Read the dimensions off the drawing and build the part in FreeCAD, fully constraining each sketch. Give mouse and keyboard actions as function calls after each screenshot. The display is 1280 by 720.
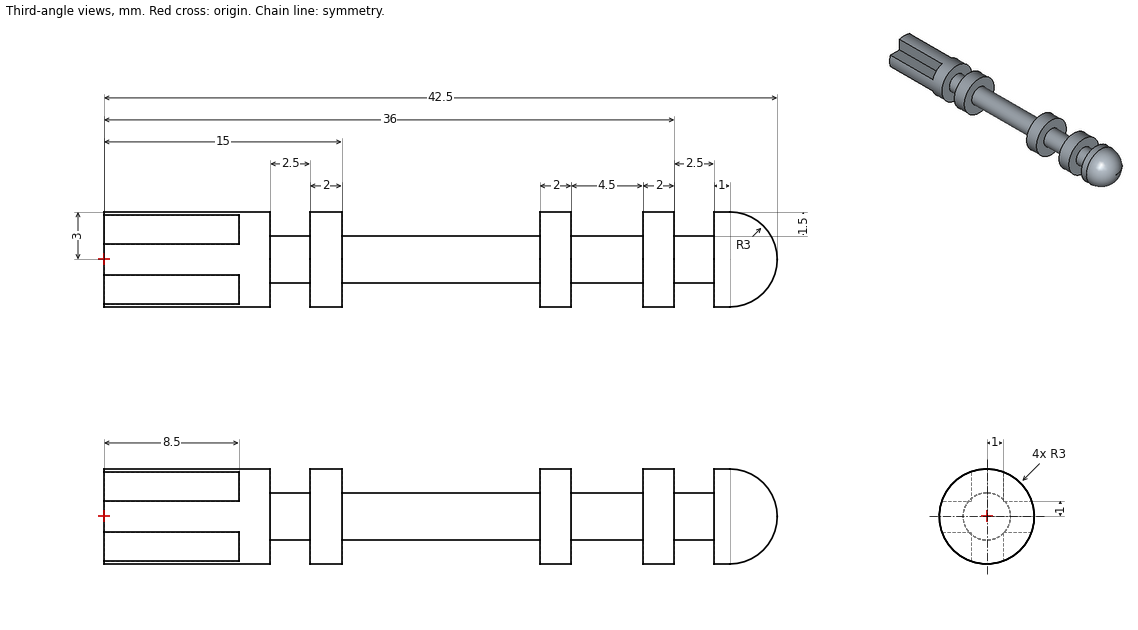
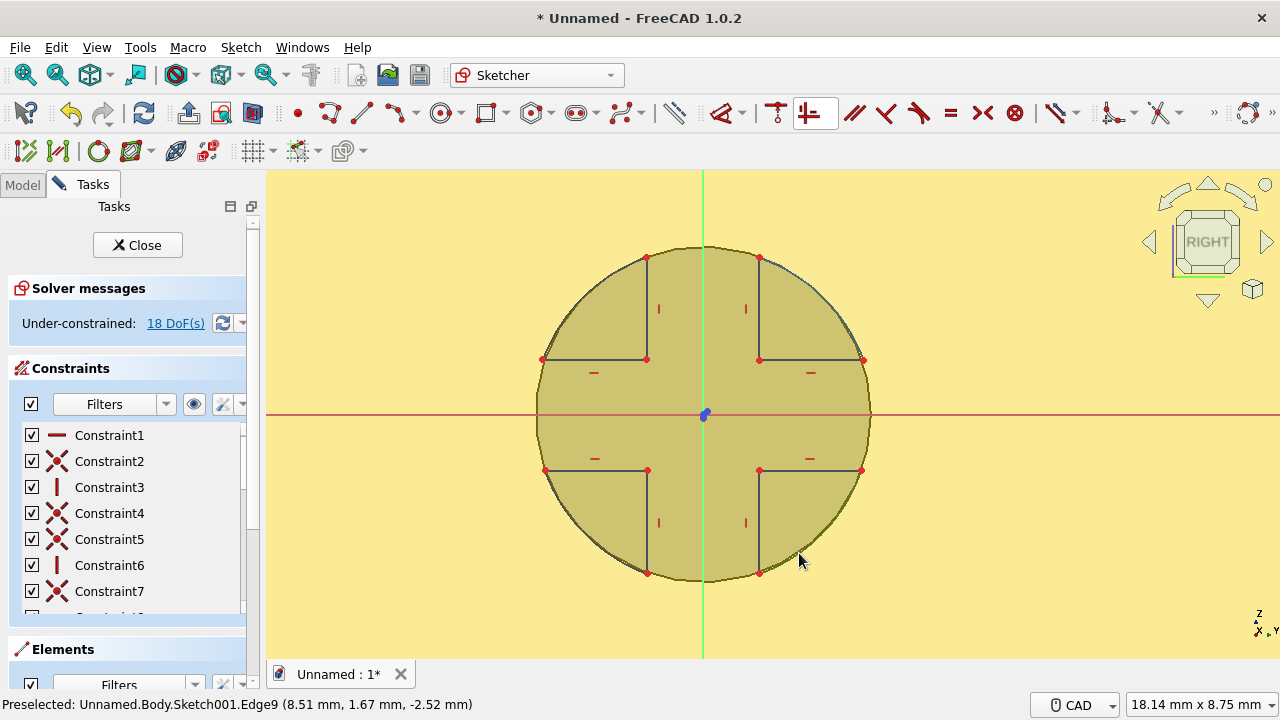
click(776, 114)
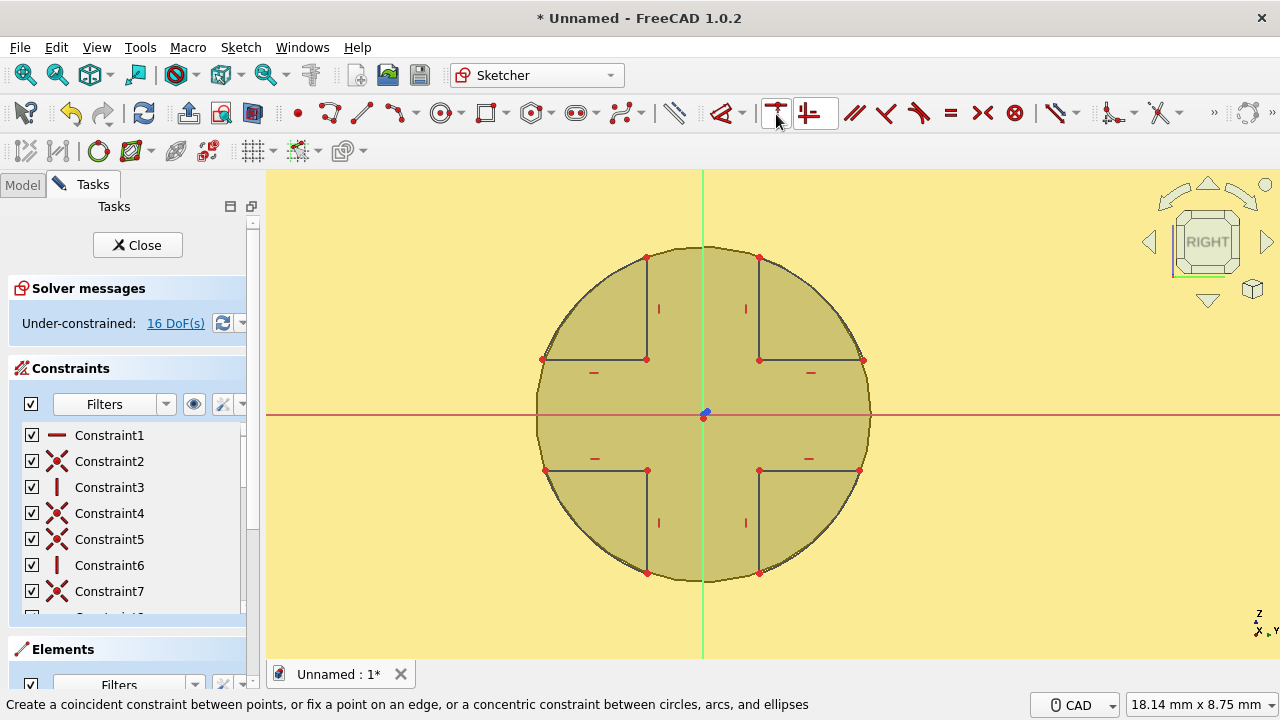
click(842, 320)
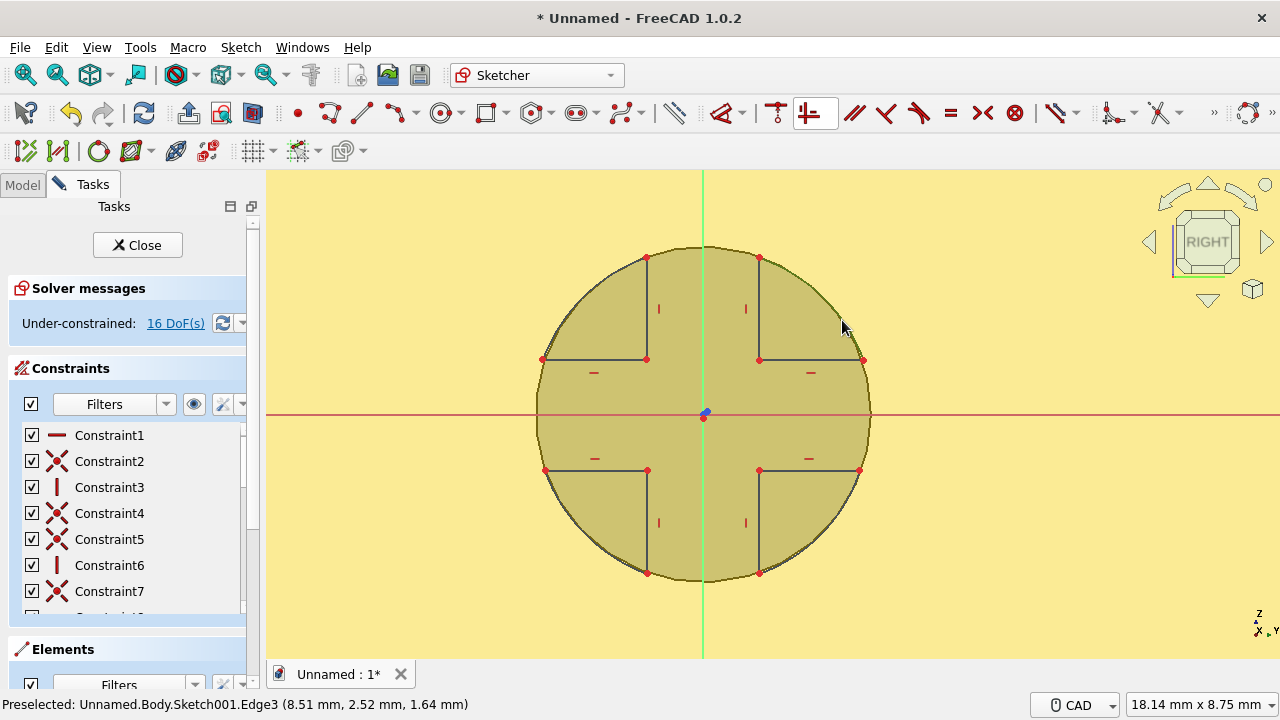
click(566, 511)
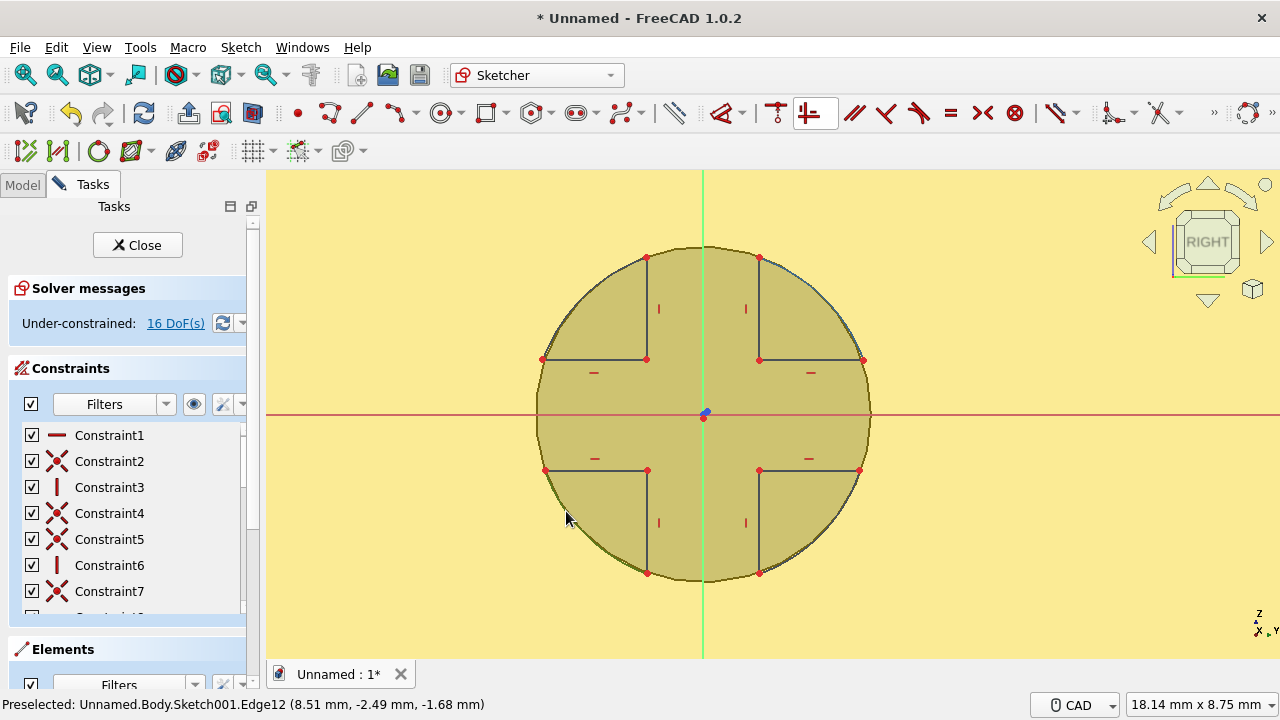
click(776, 114)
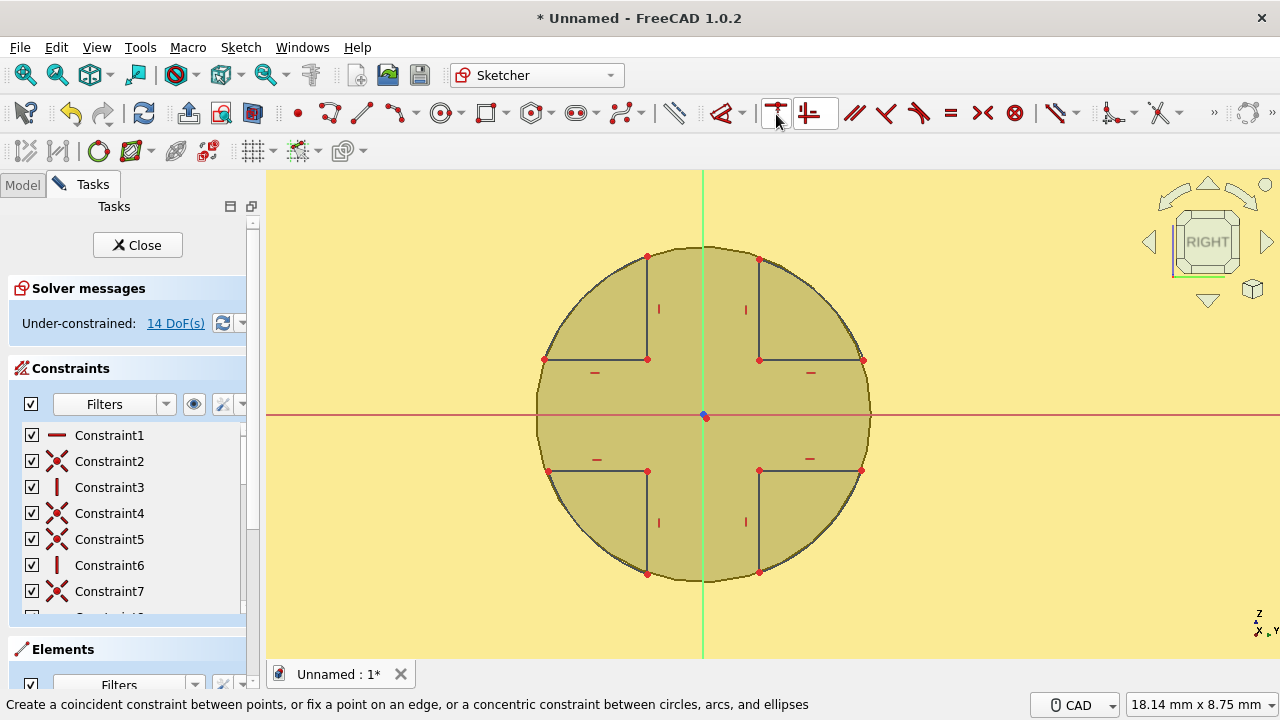
drag(693, 404, 717, 428)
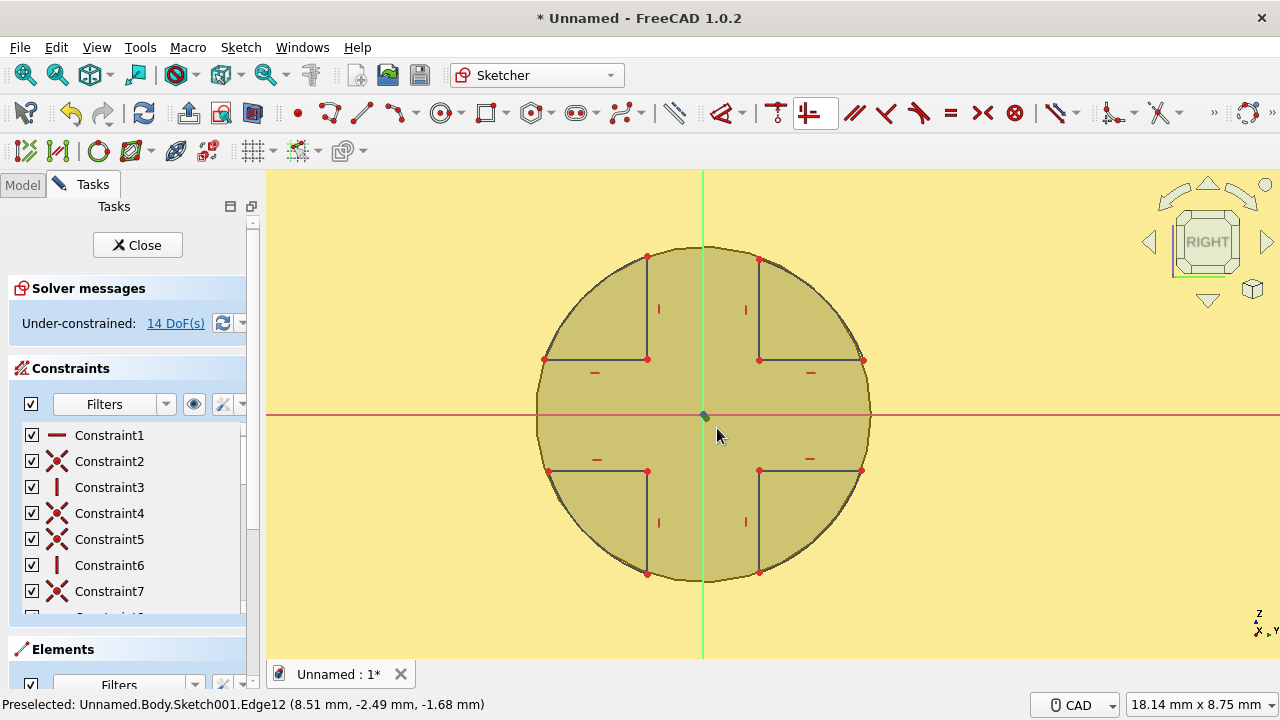
click(776, 114)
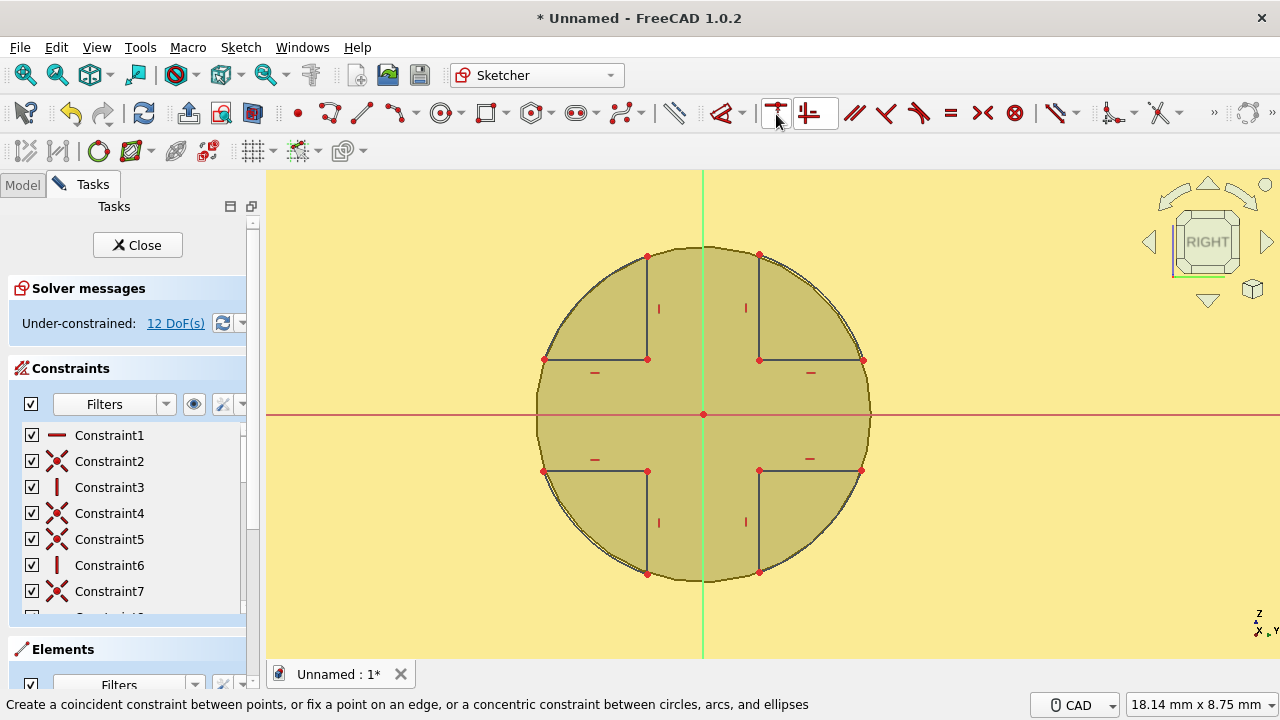
click(843, 319)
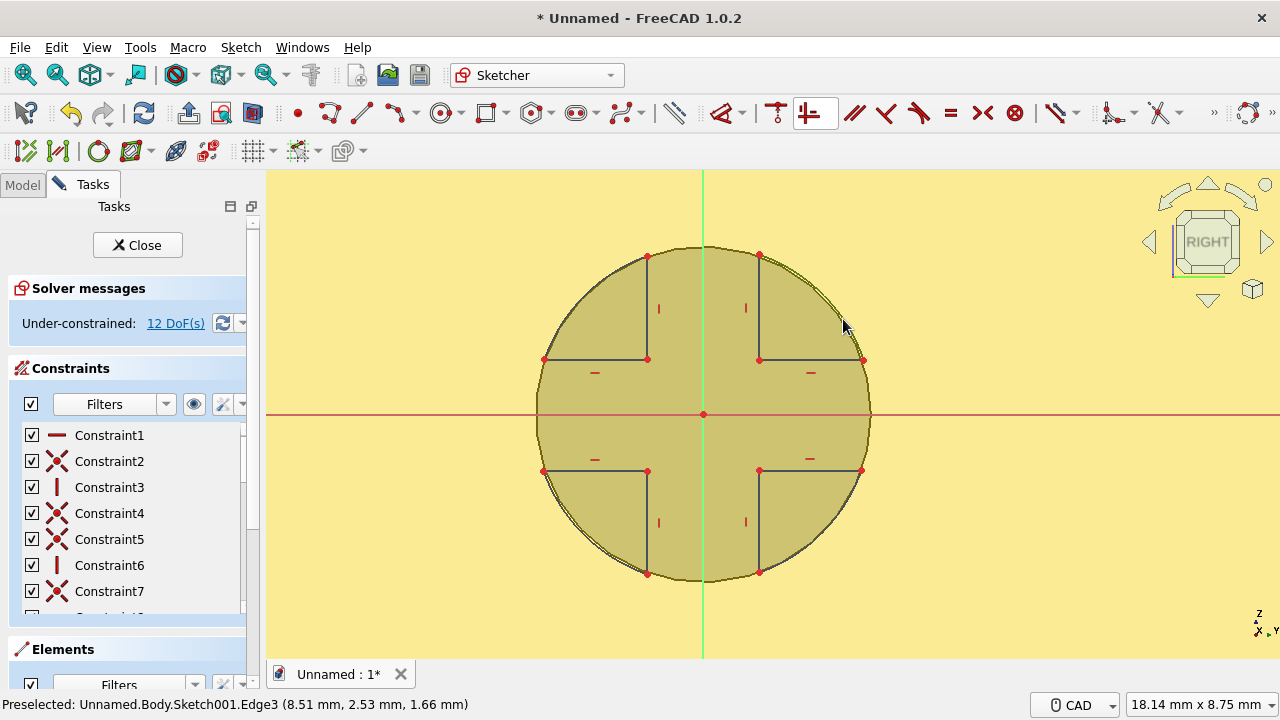
click(607, 277)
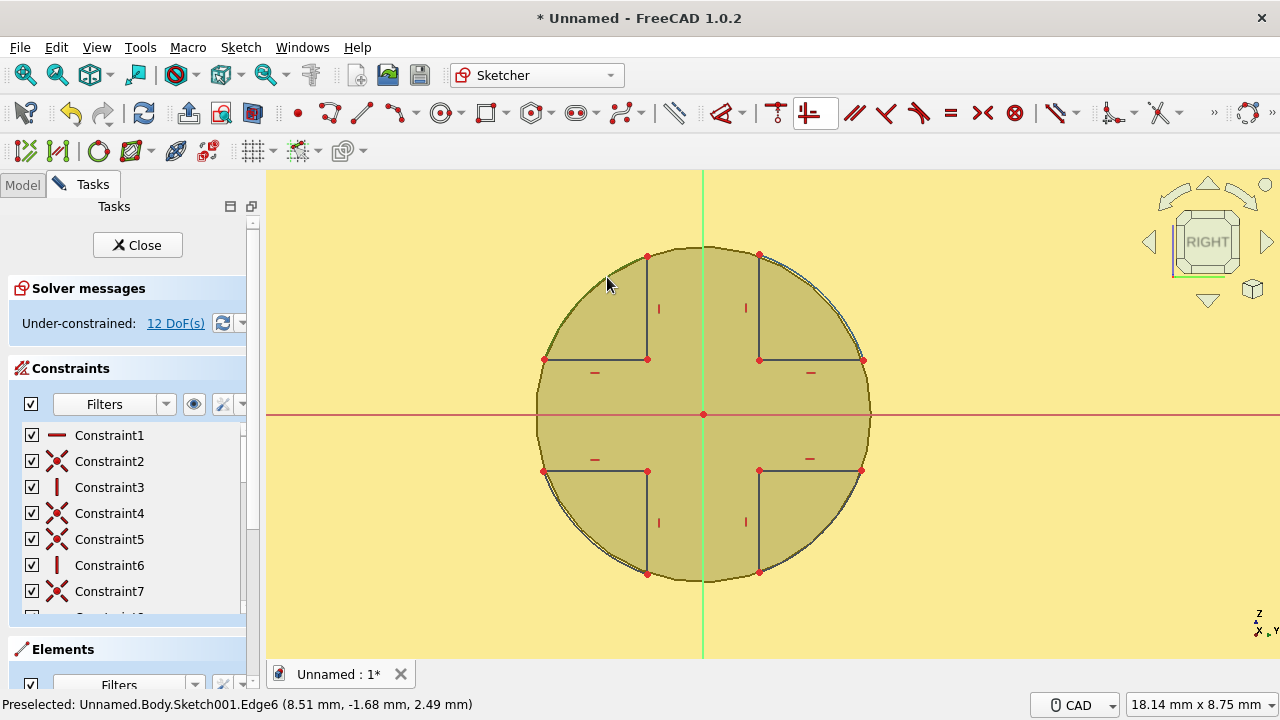
click(799, 552)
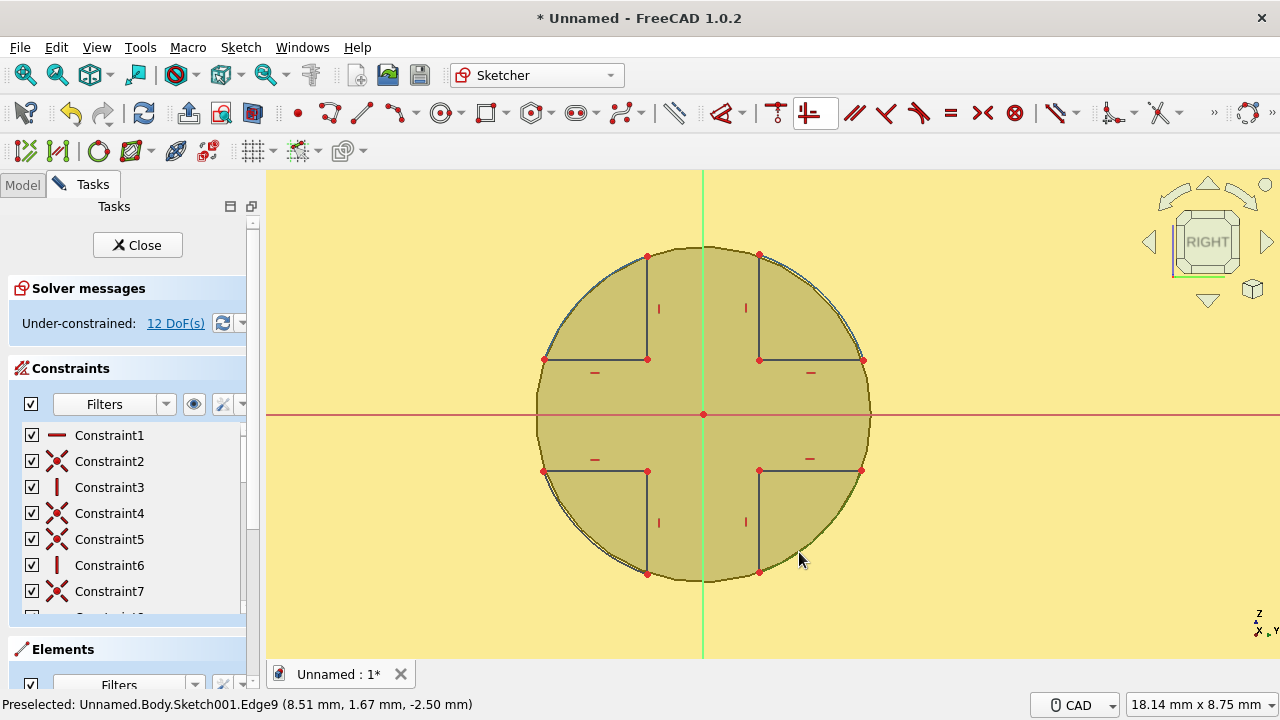
click(564, 511)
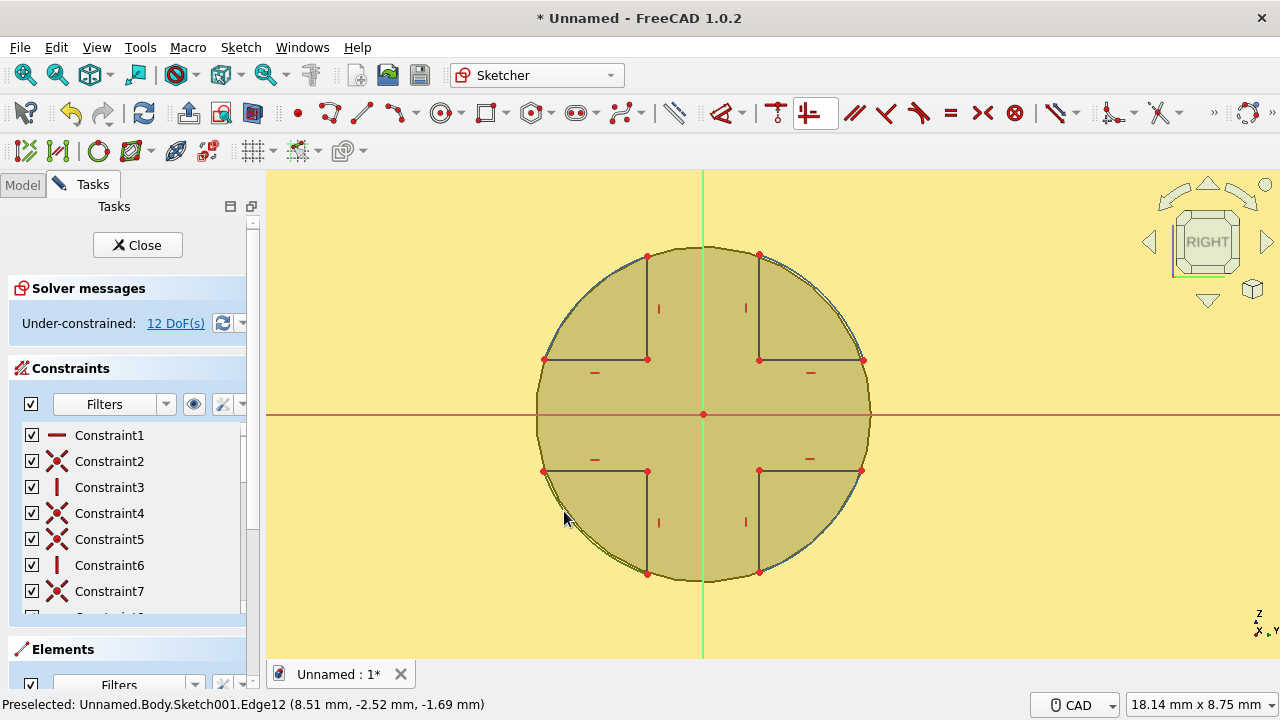
click(952, 114)